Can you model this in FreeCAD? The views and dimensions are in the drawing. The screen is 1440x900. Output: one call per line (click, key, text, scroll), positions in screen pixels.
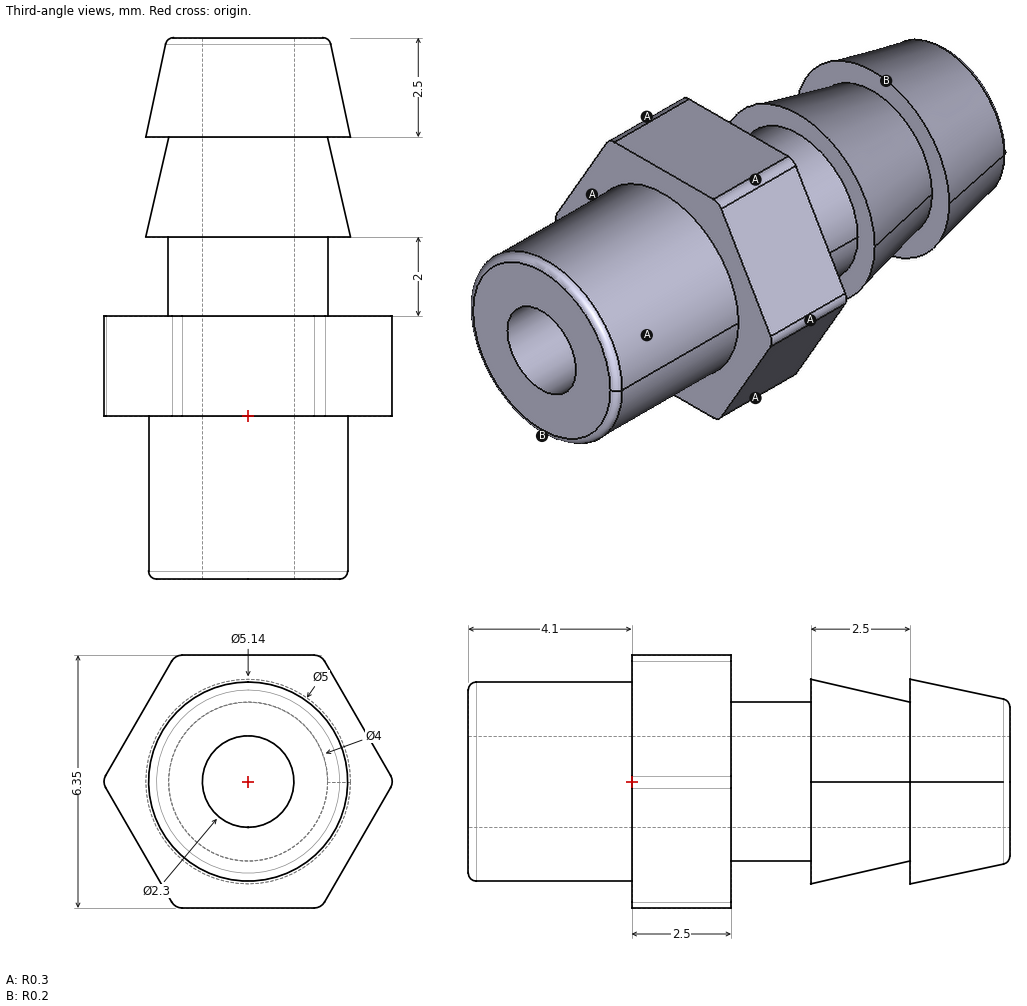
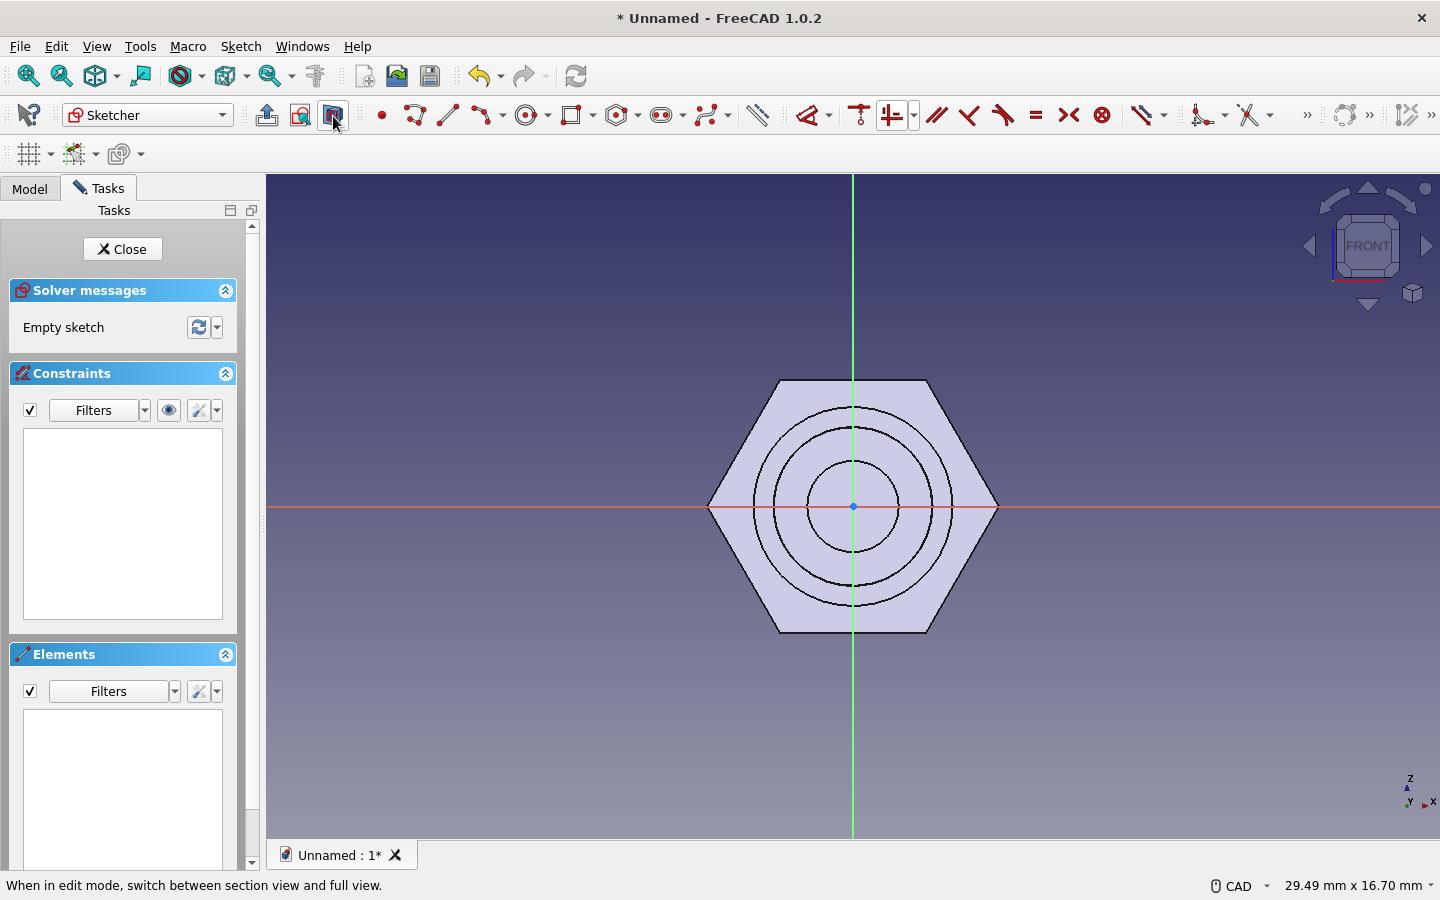
scroll(870, 507, up, 8)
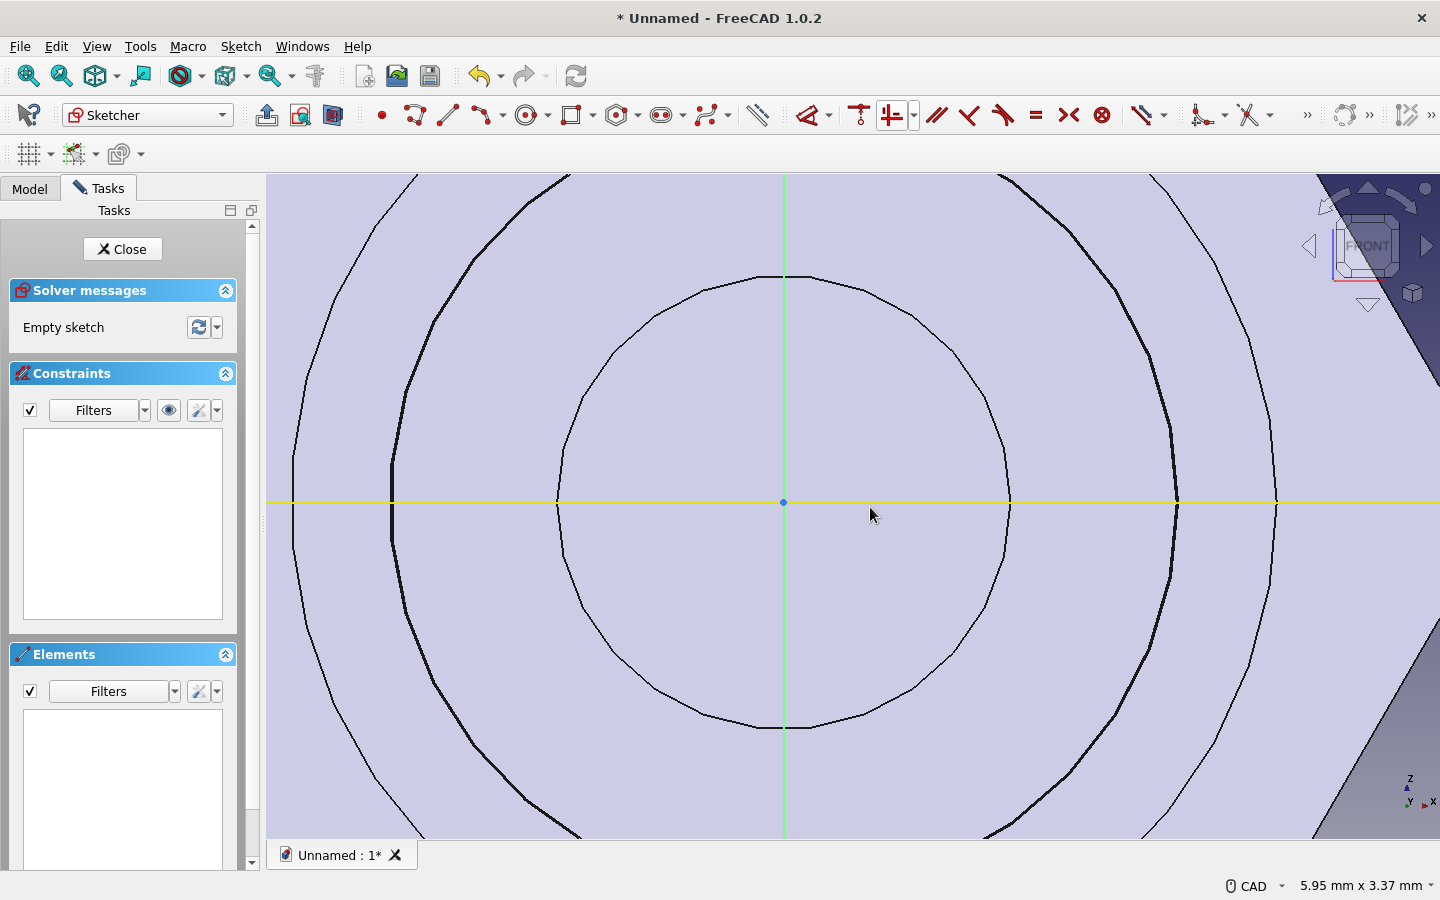
click(526, 116)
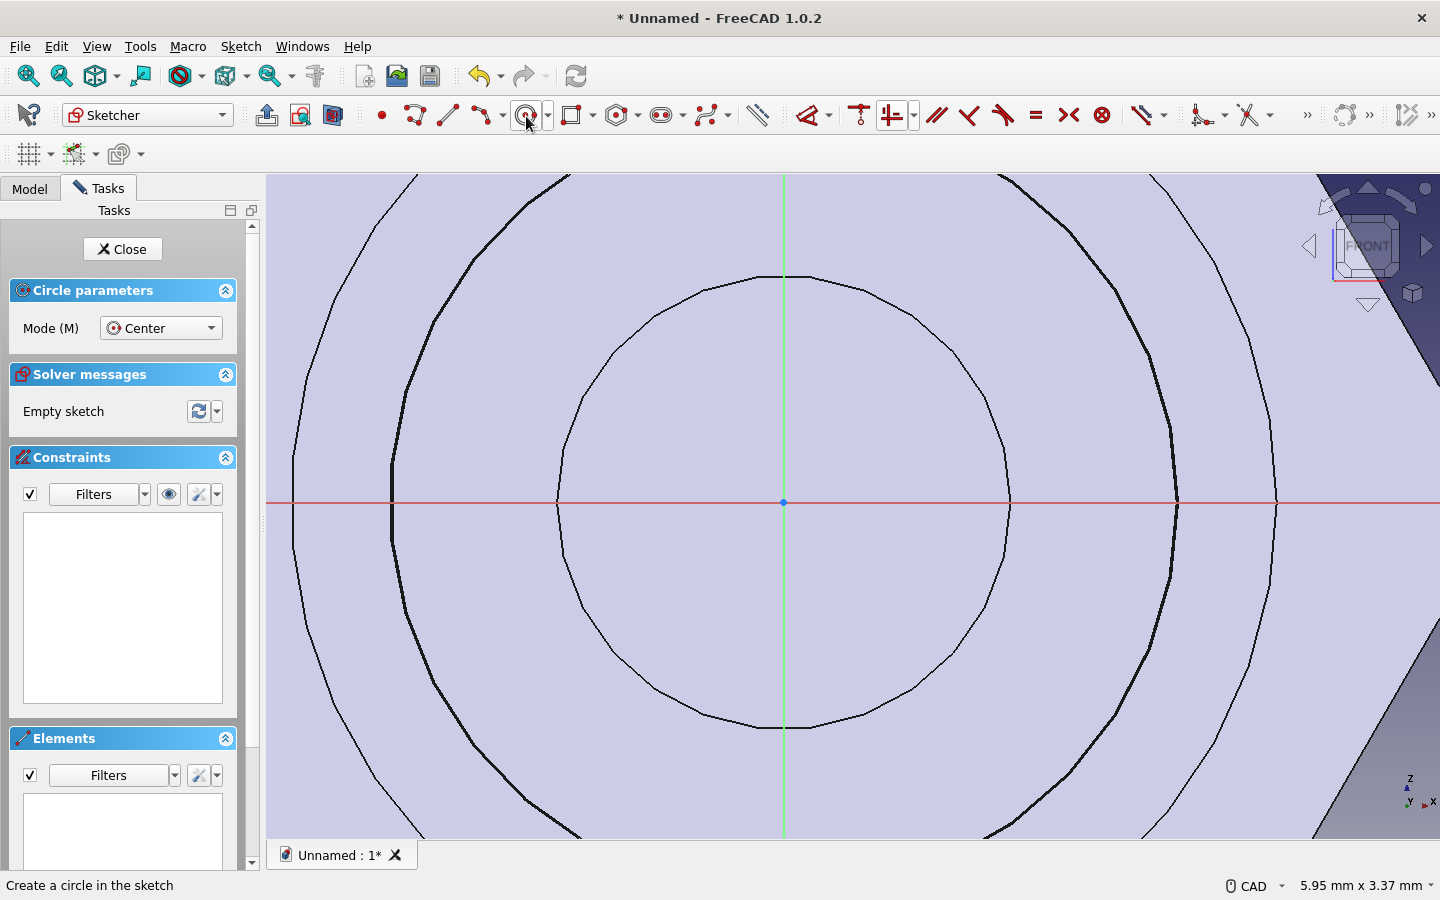
click(784, 503)
click(944, 342)
key(Escape)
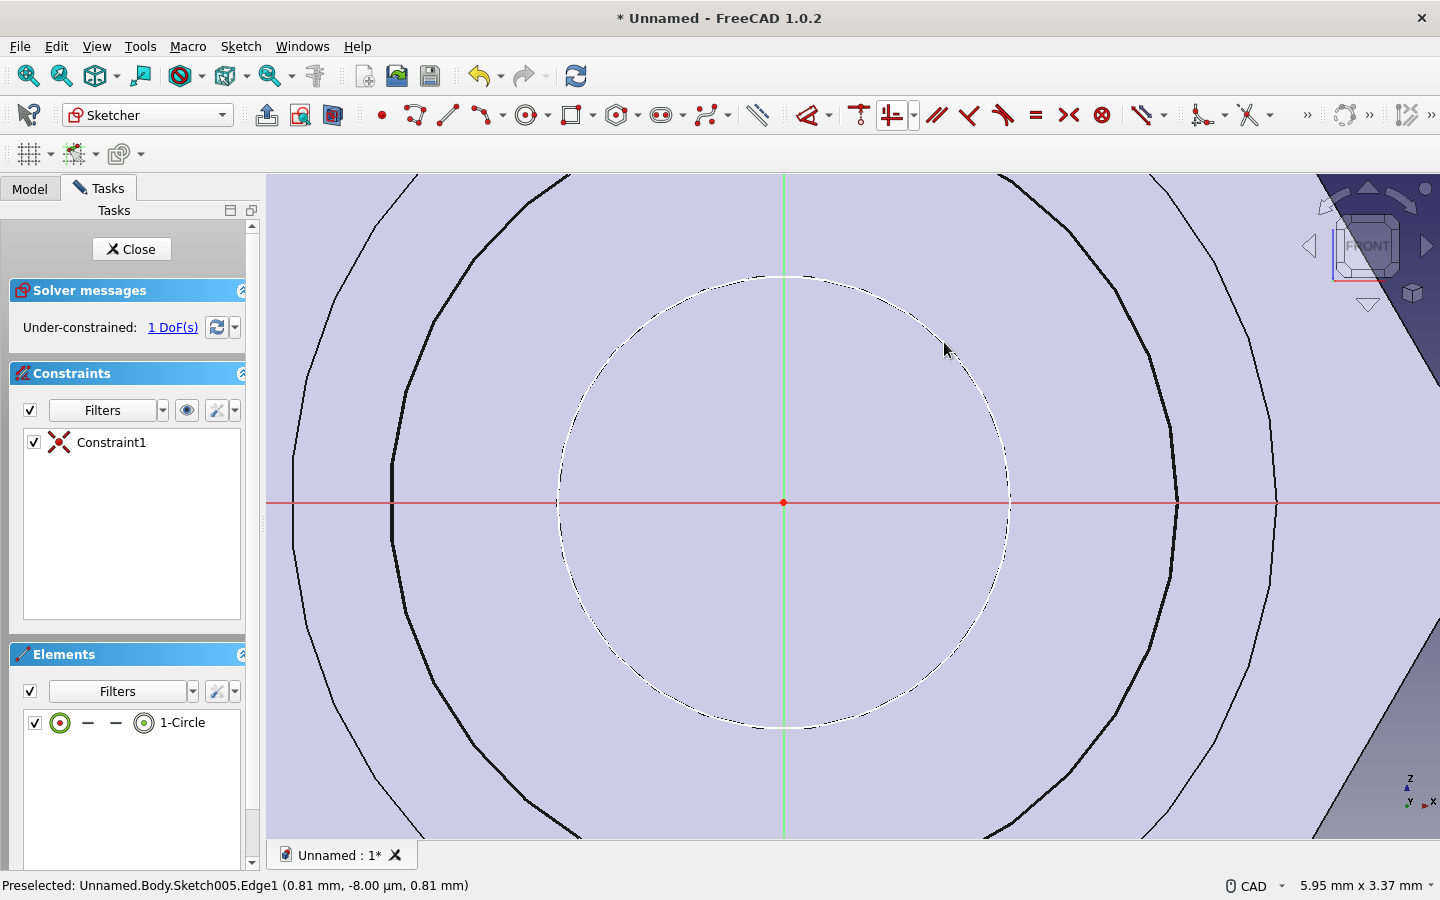
key(d)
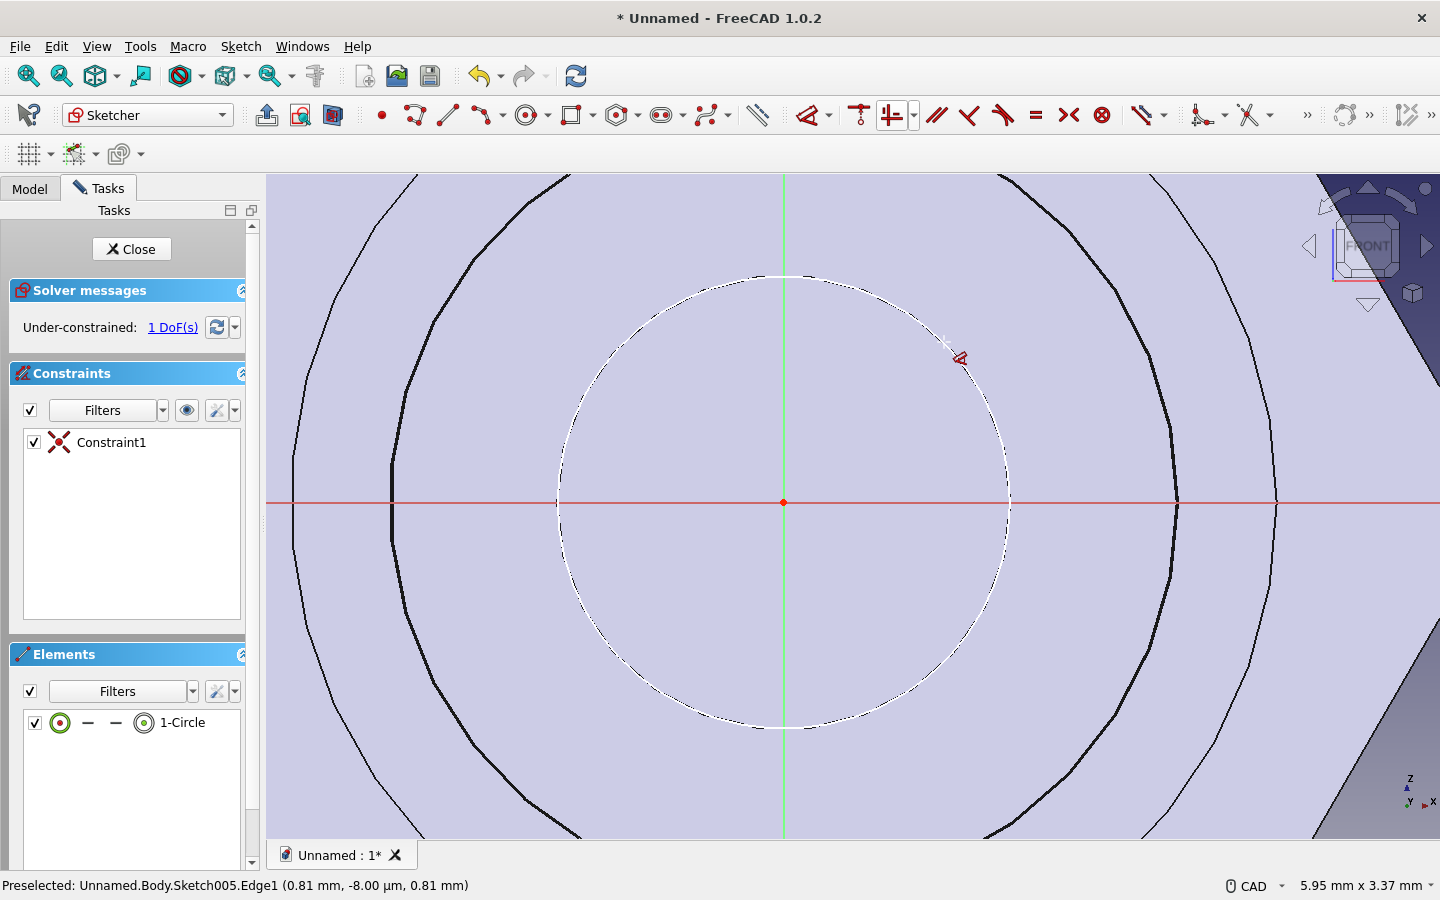
click(943, 342)
click(966, 319)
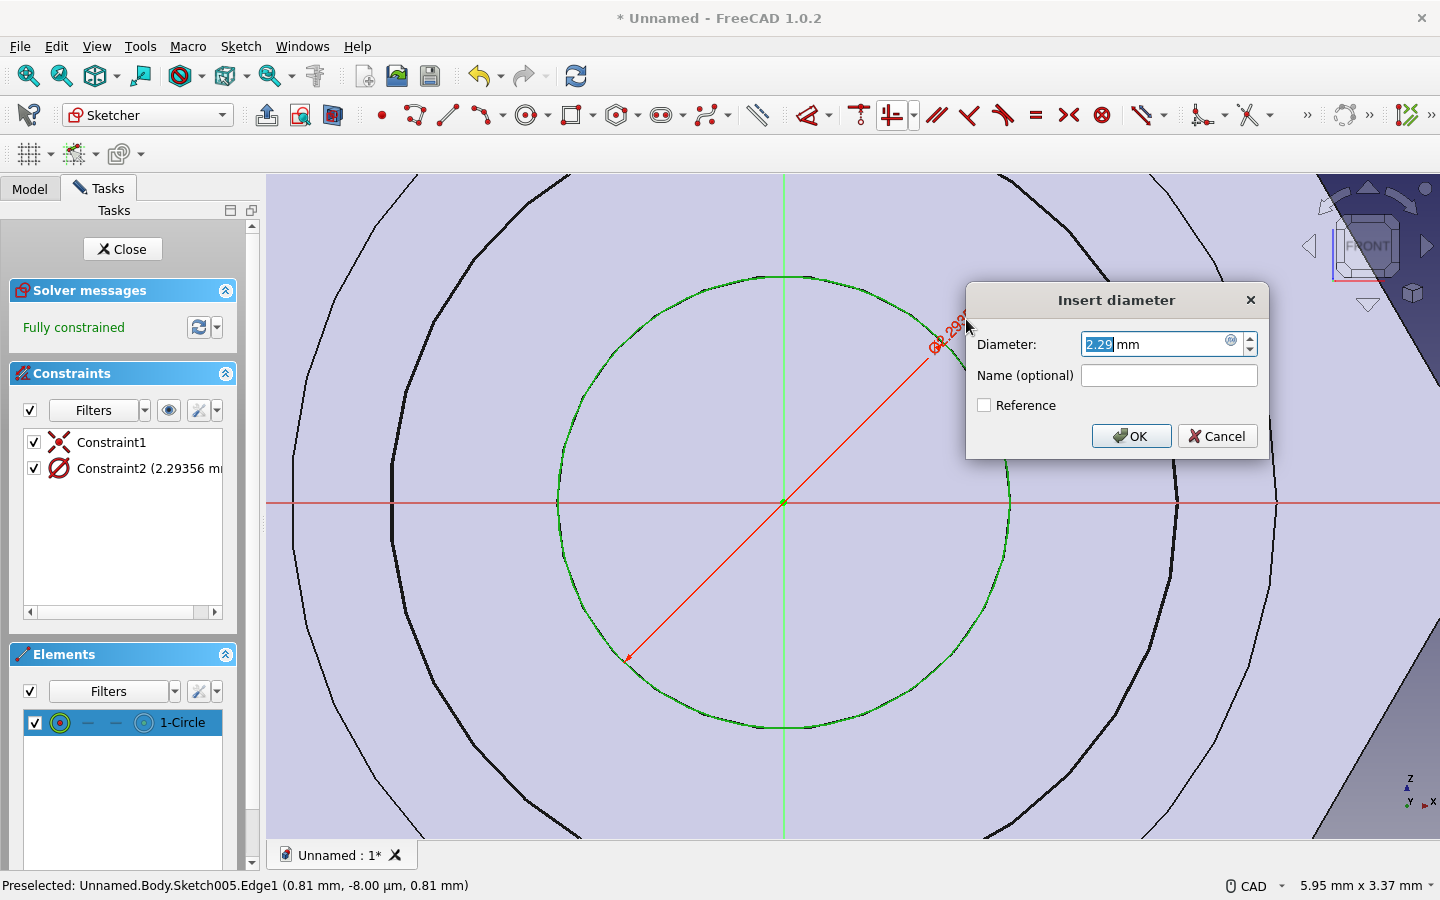
text(2.3)
key(Return)
key(Escape)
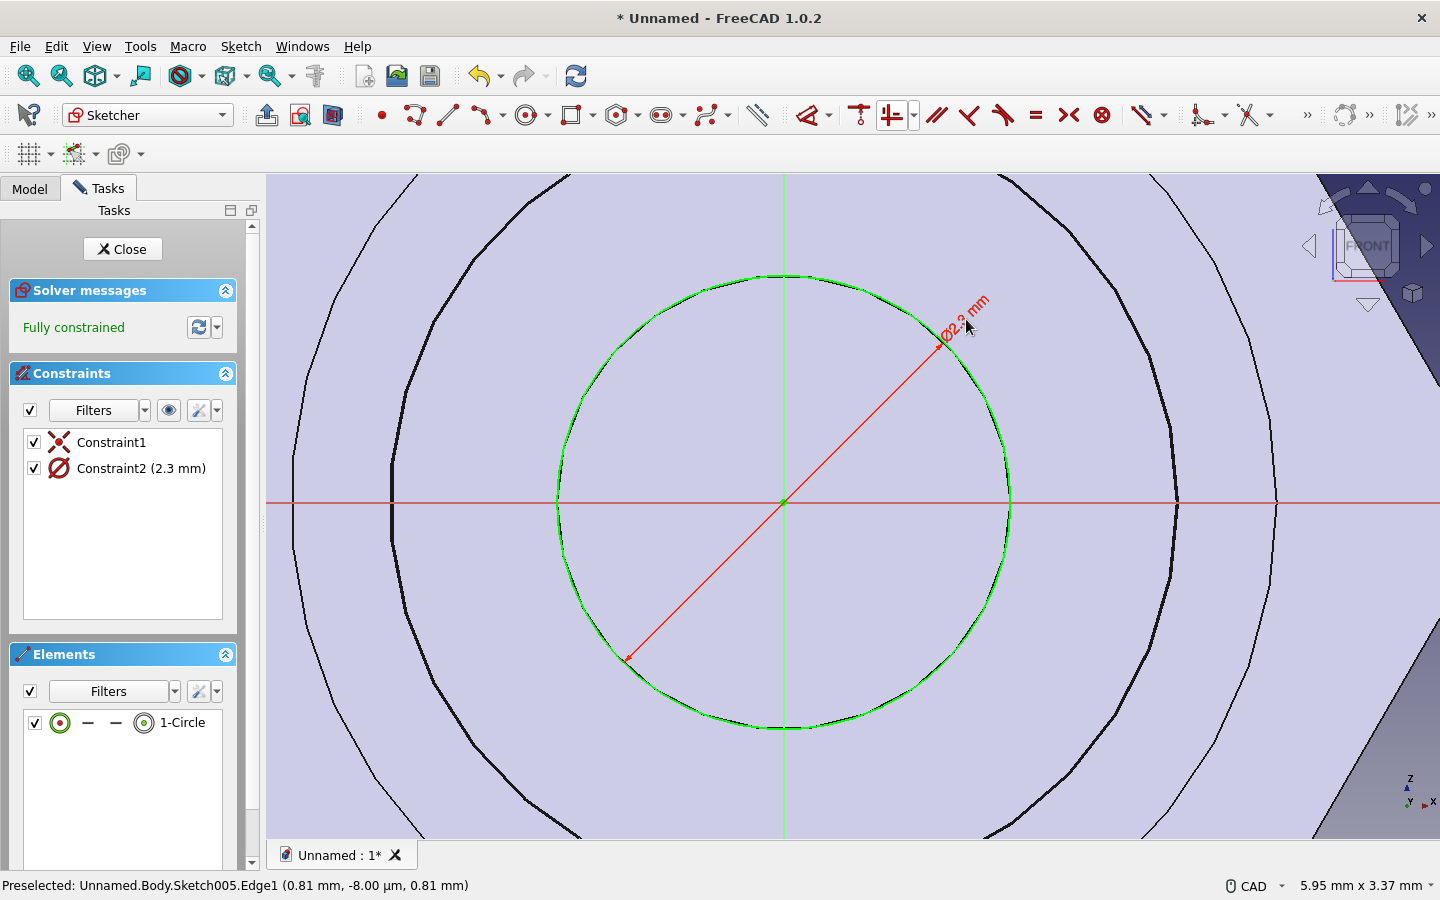
click(123, 249)